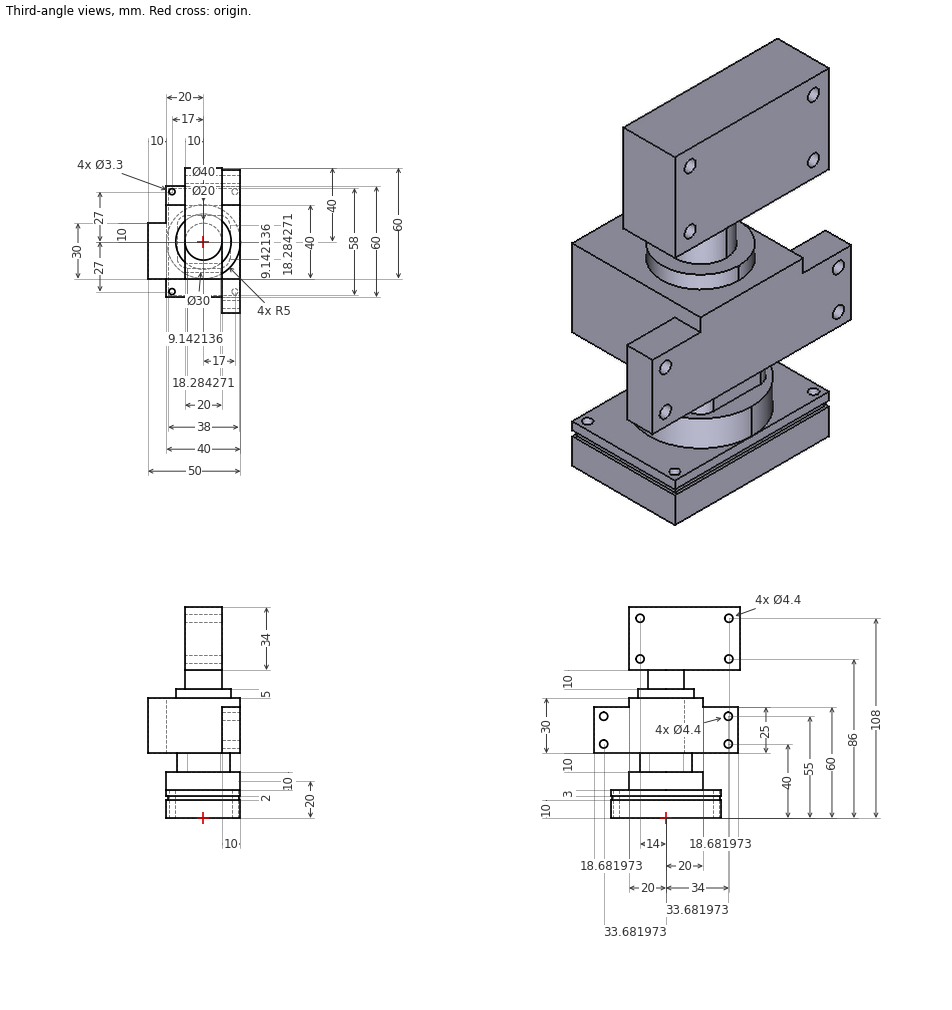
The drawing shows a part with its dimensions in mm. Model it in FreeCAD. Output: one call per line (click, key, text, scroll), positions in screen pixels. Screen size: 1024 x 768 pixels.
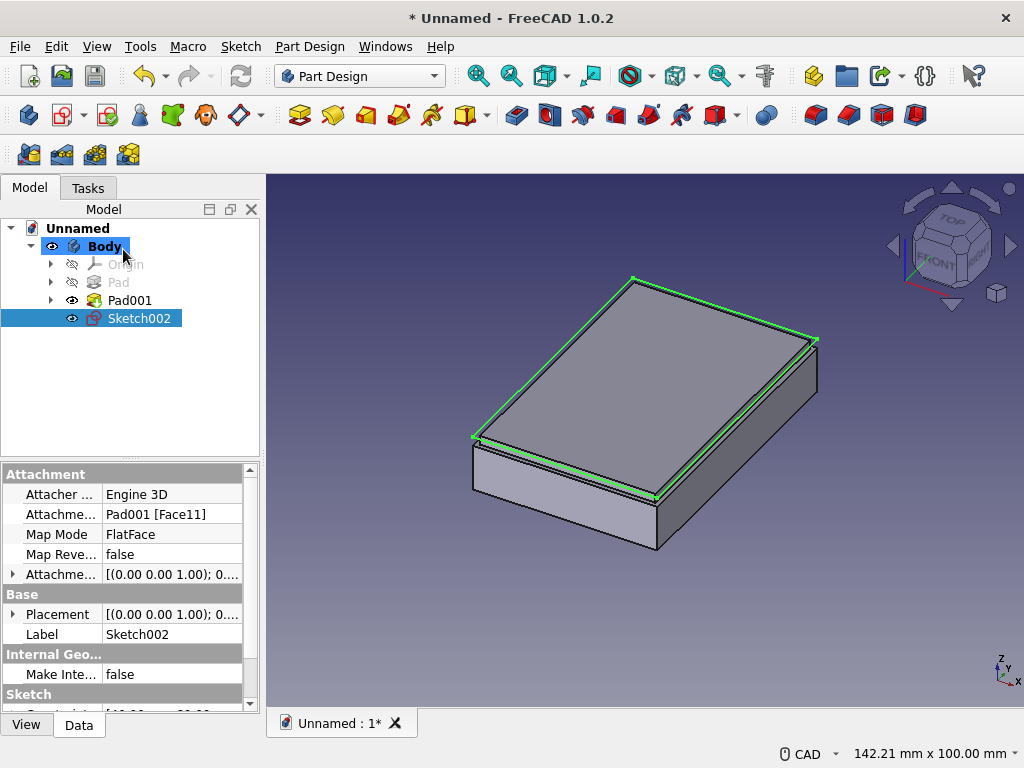
click(300, 116)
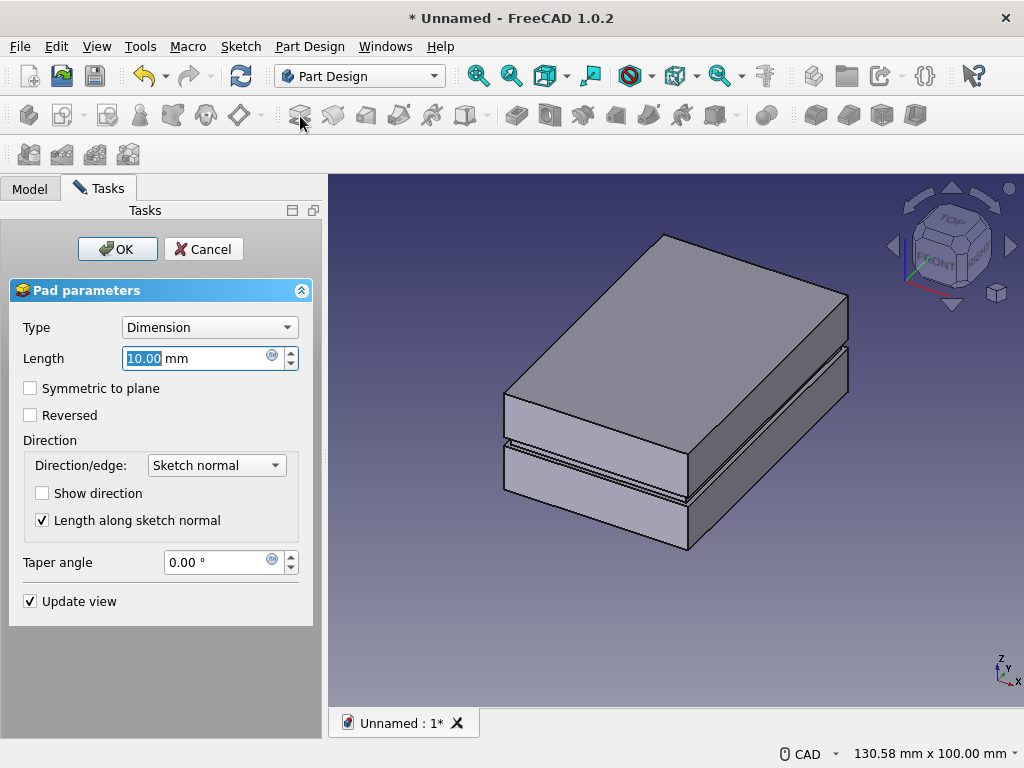
text(3)
key(Tab)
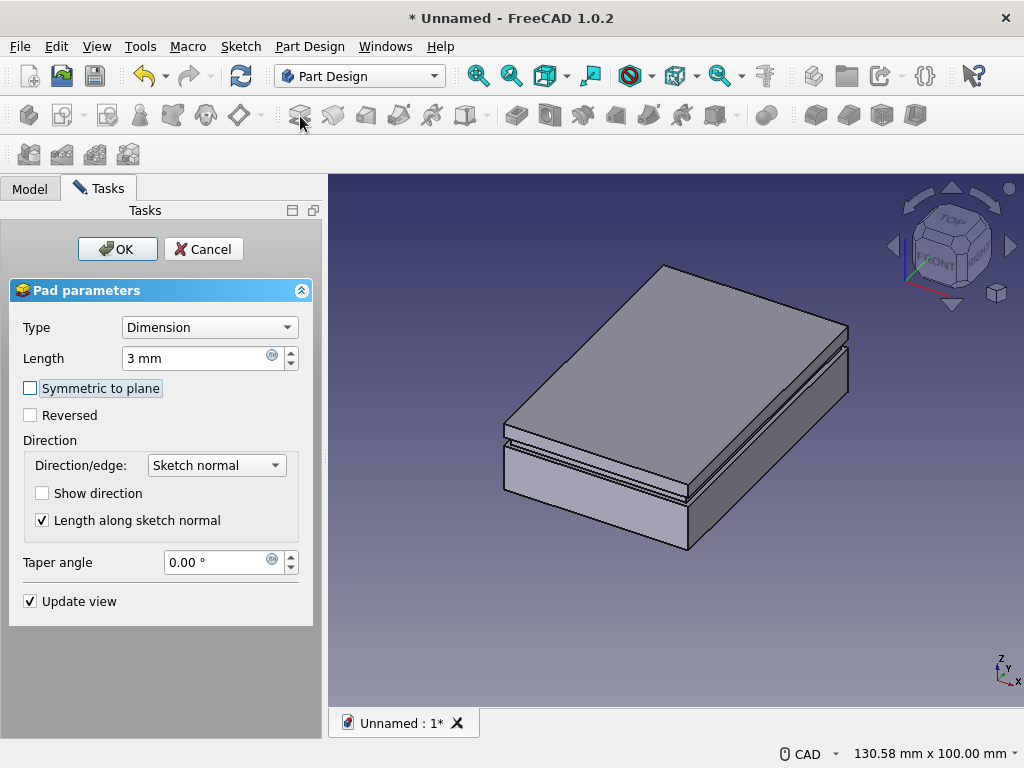
click(118, 249)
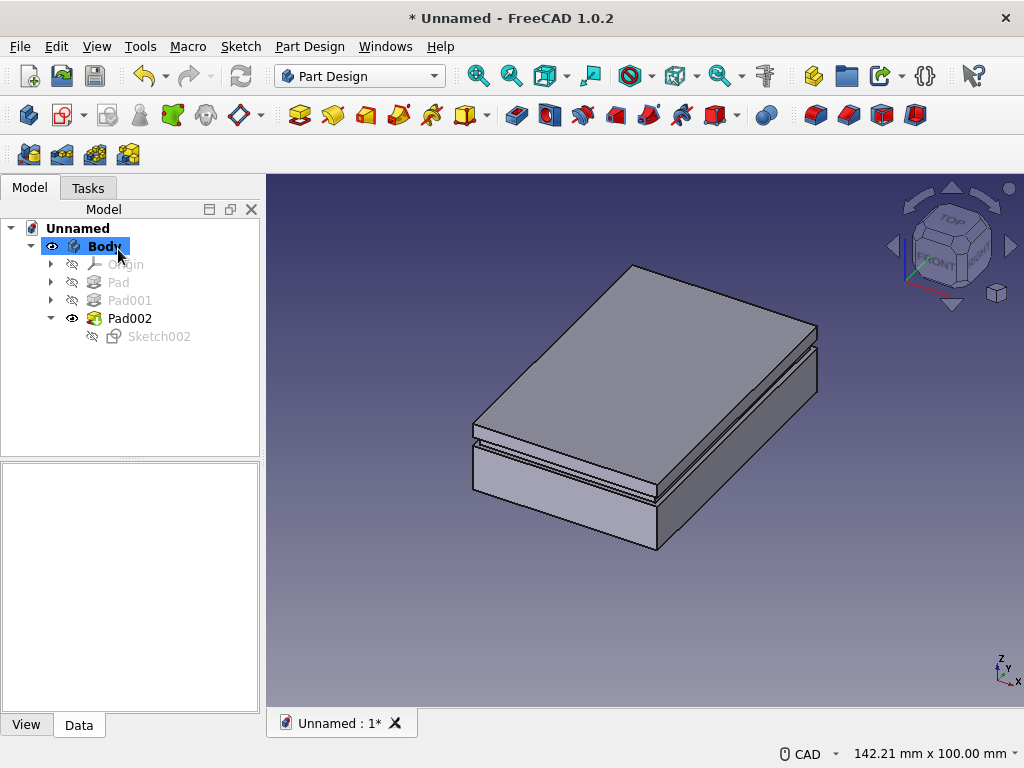
click(668, 351)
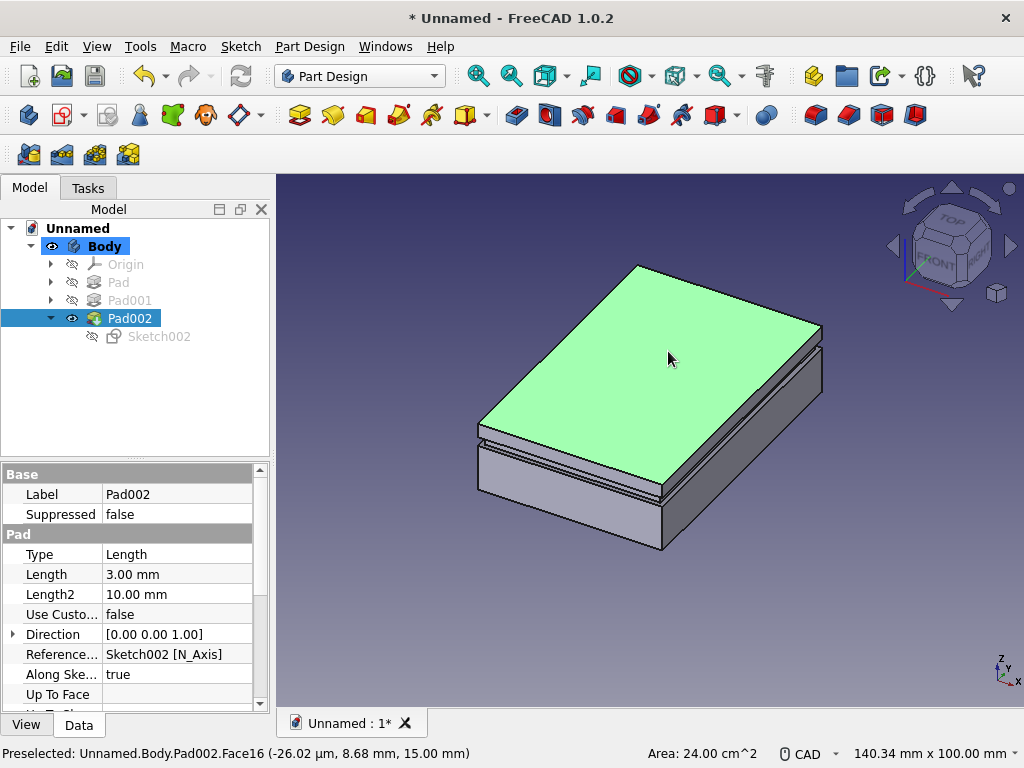
click(62, 116)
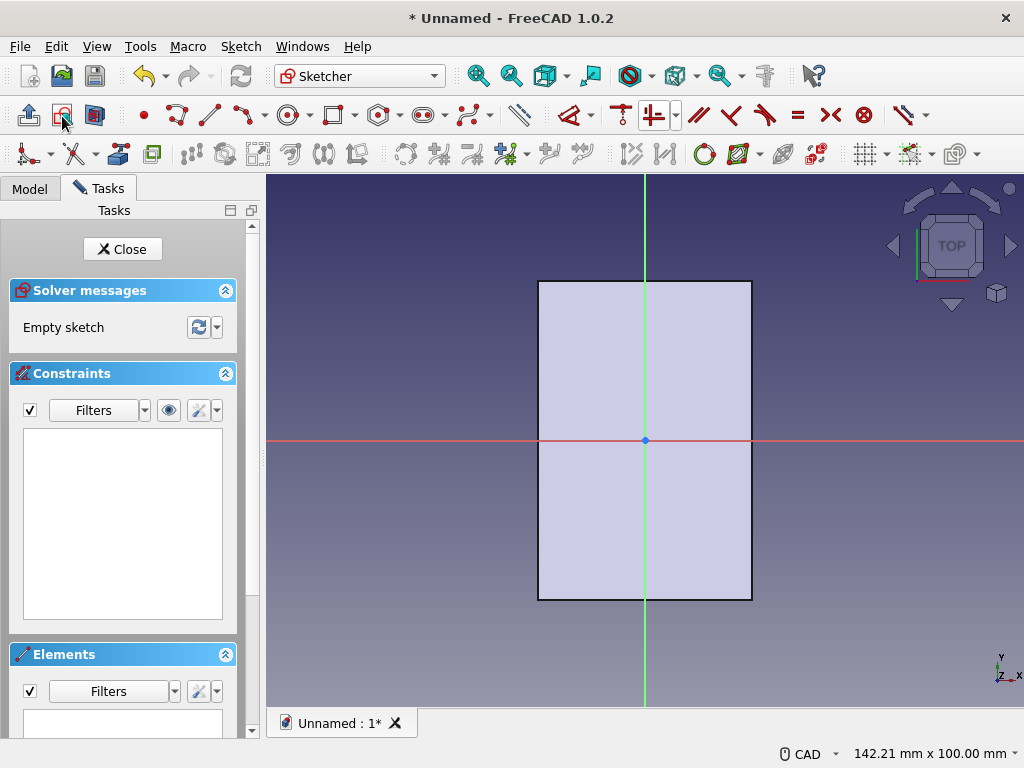
scroll(784, 440, up, 2)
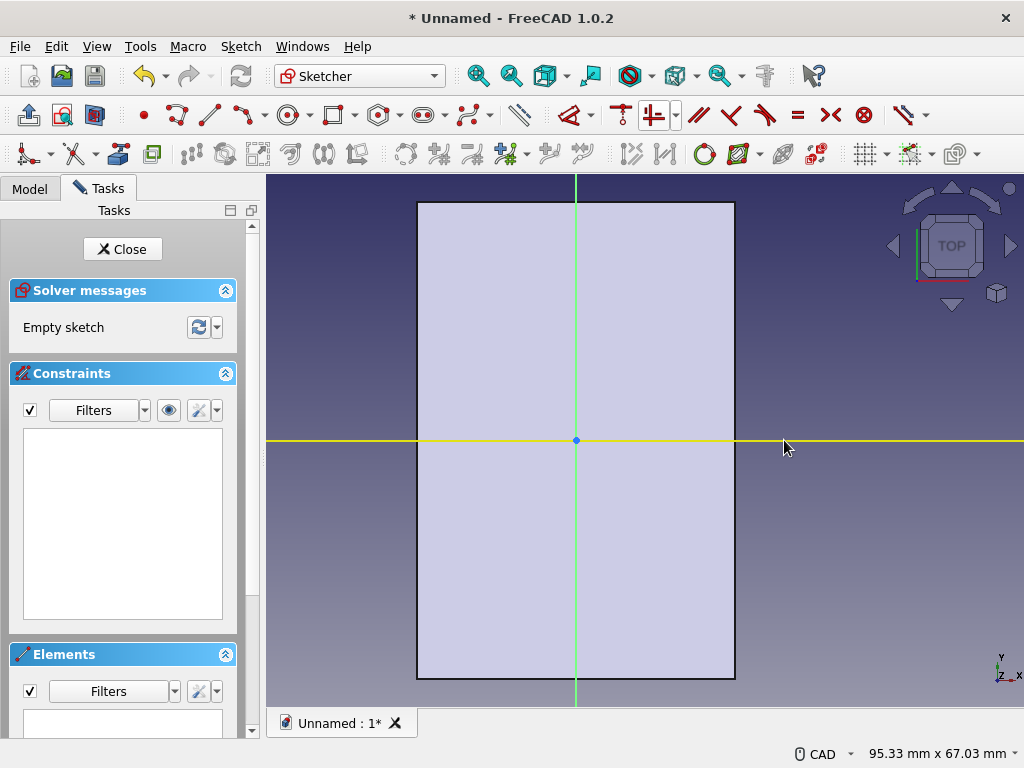
key(g)
key(c)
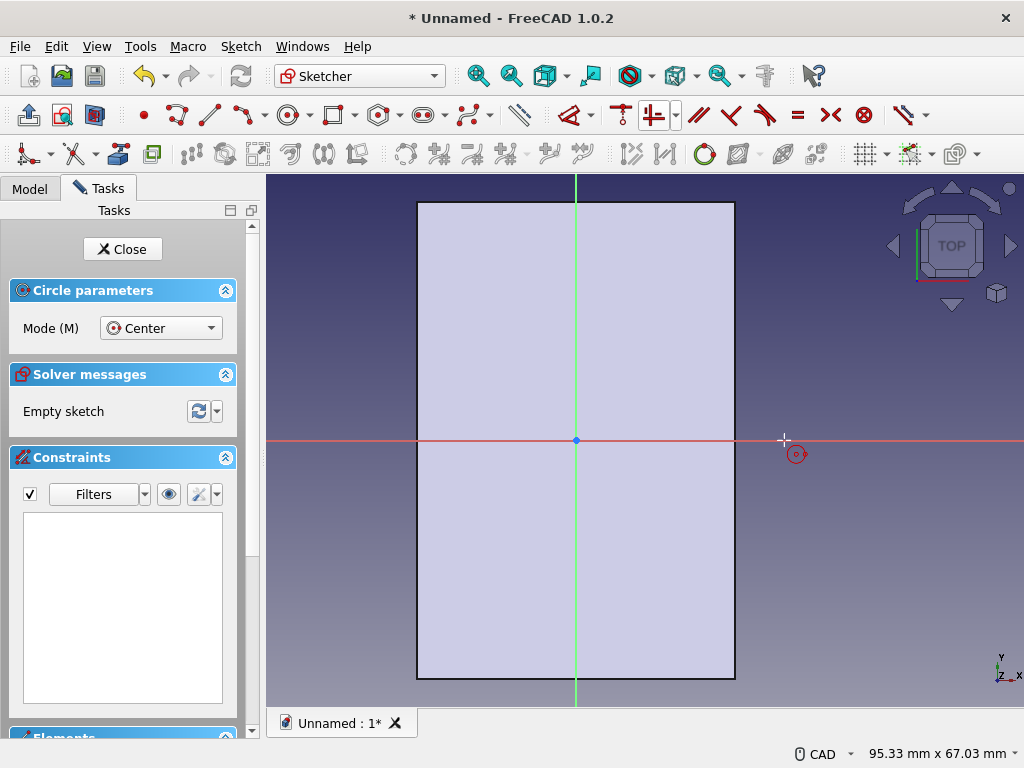
click(576, 440)
move(689, 328)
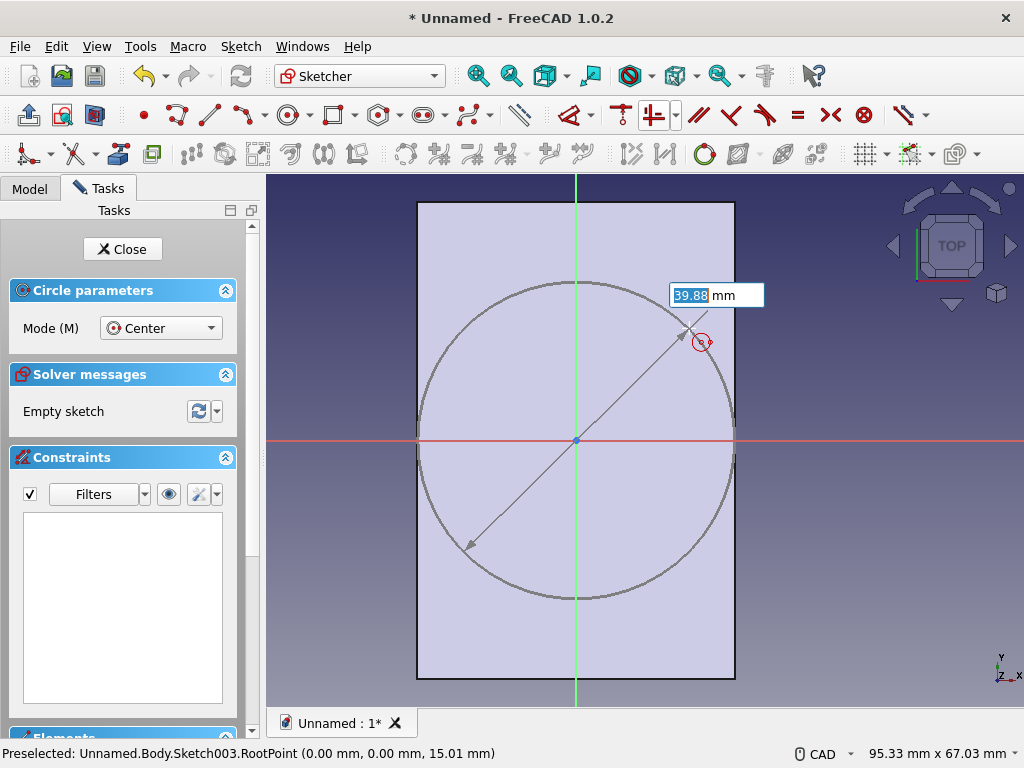
text(40)
key(Return)
key(Escape)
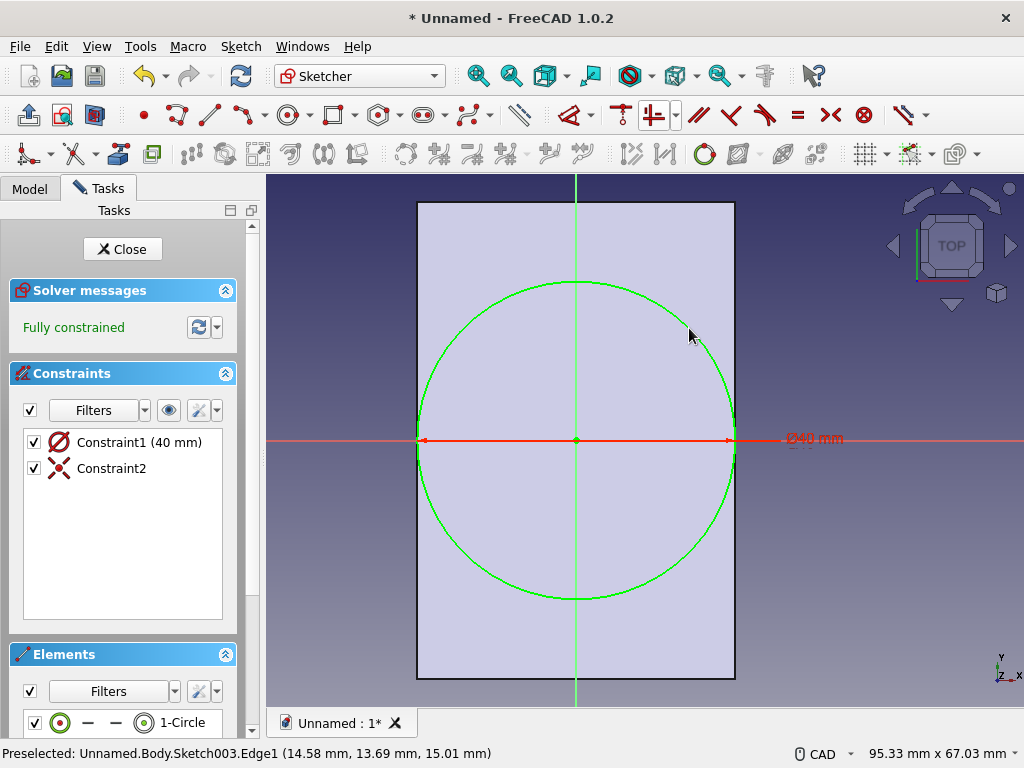
click(123, 249)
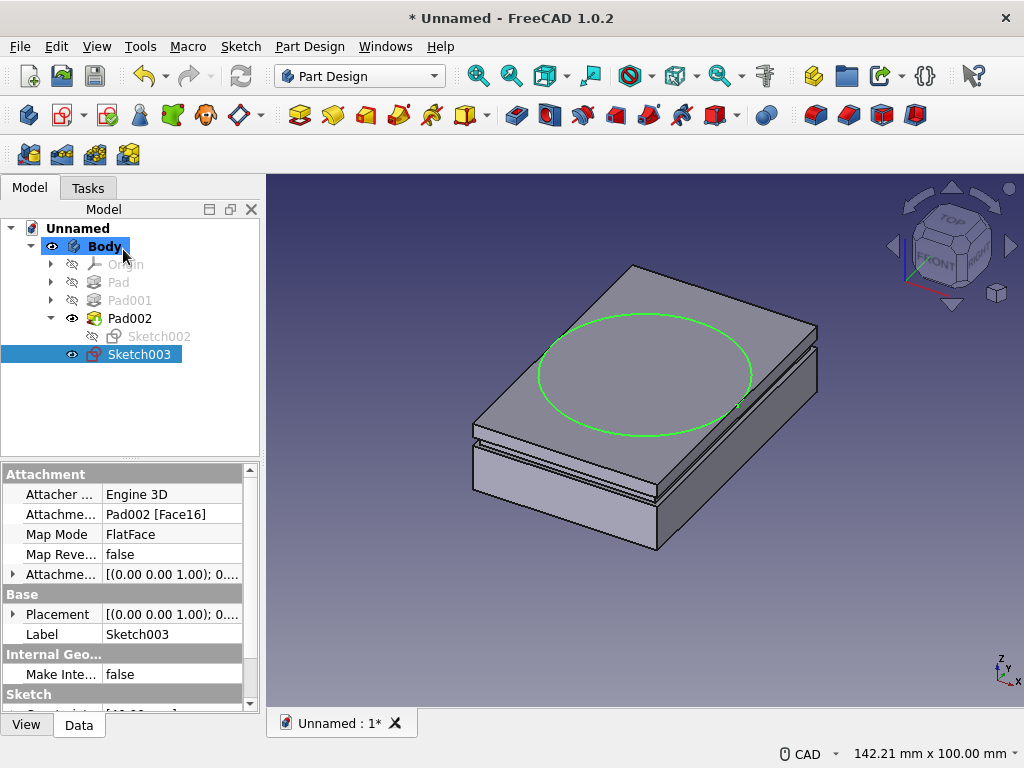
click(300, 116)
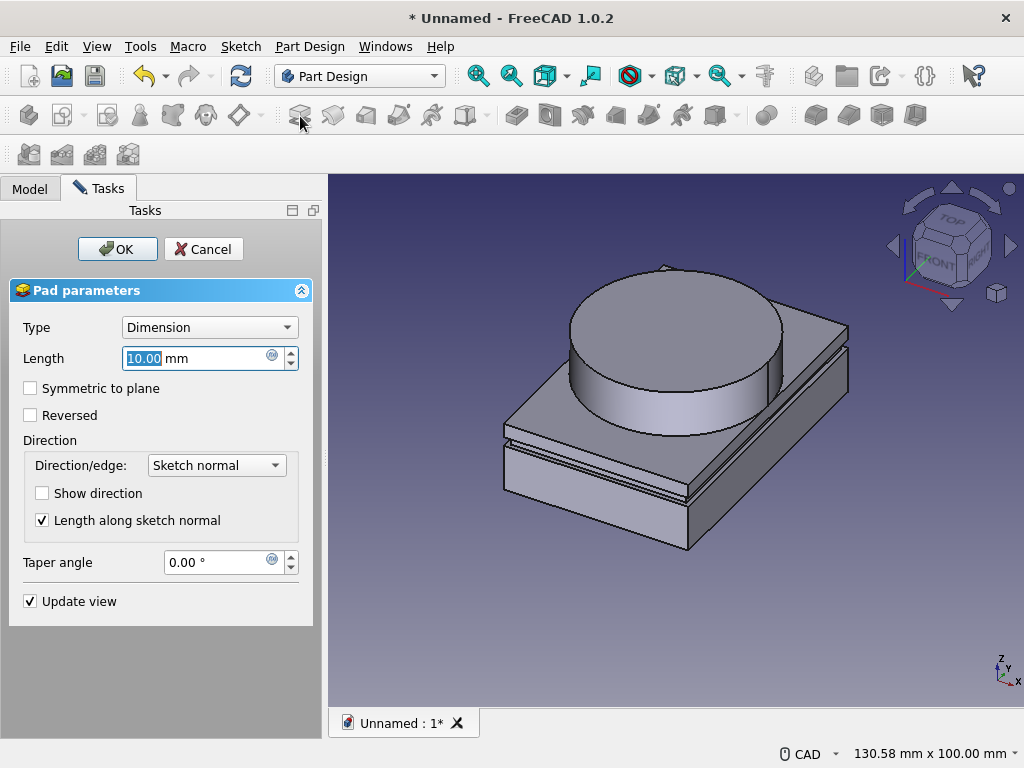
text(10)
key(Tab)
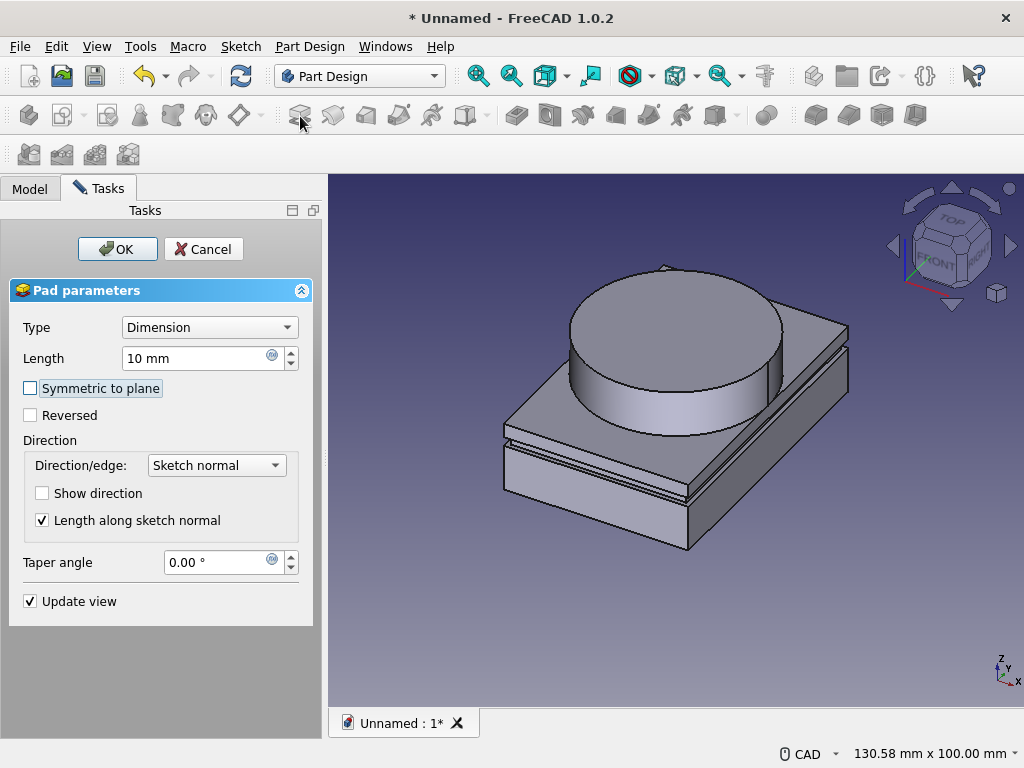
click(118, 249)